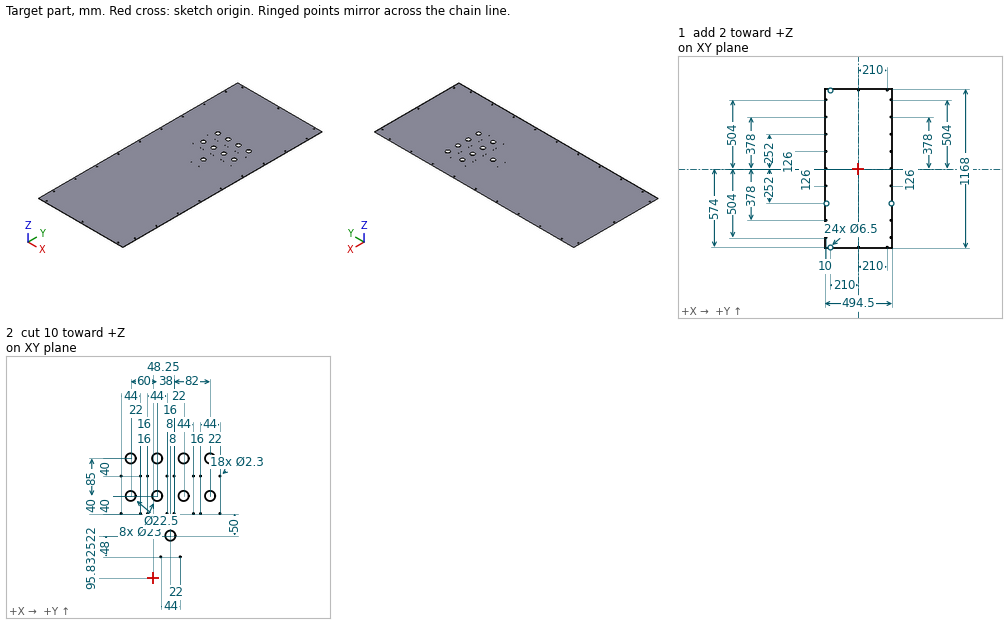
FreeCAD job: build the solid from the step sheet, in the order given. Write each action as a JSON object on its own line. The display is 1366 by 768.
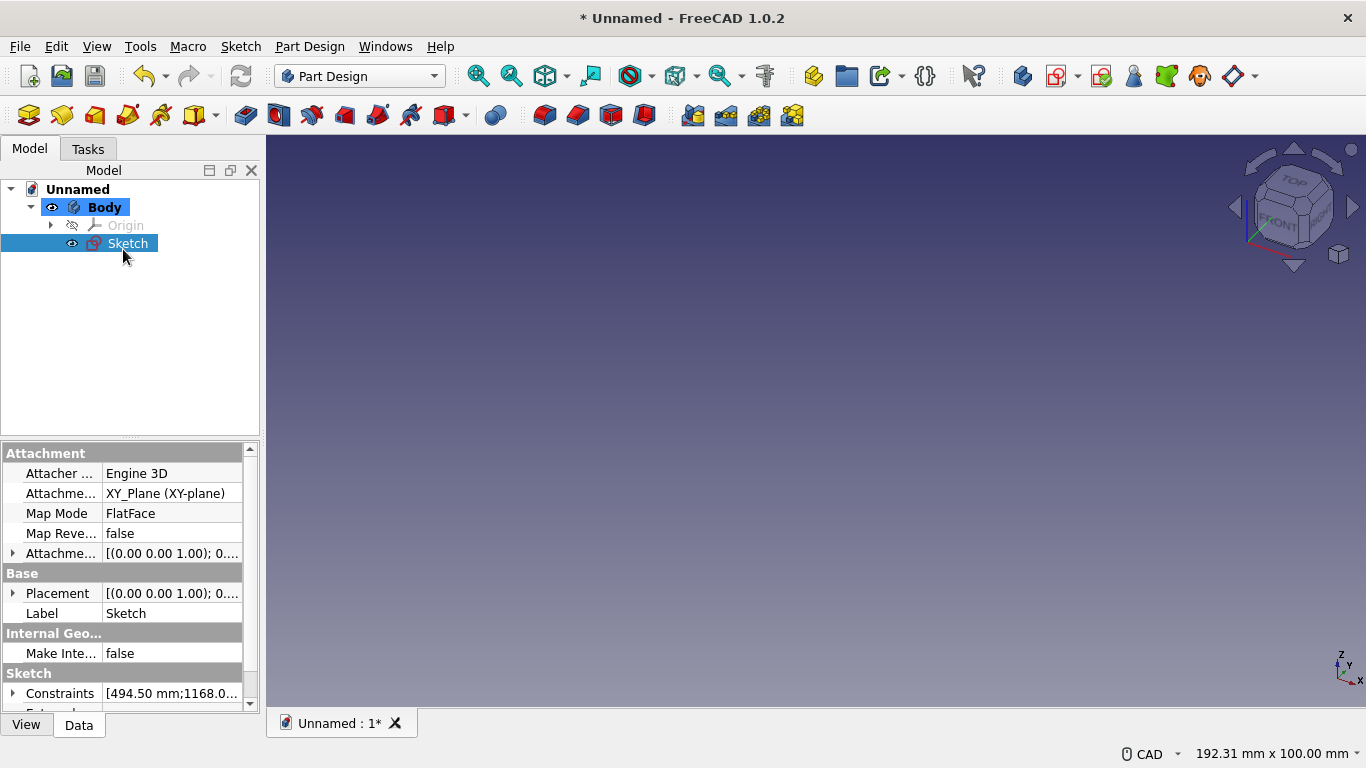
{"action": "left_click", "coordinate": [29, 116]}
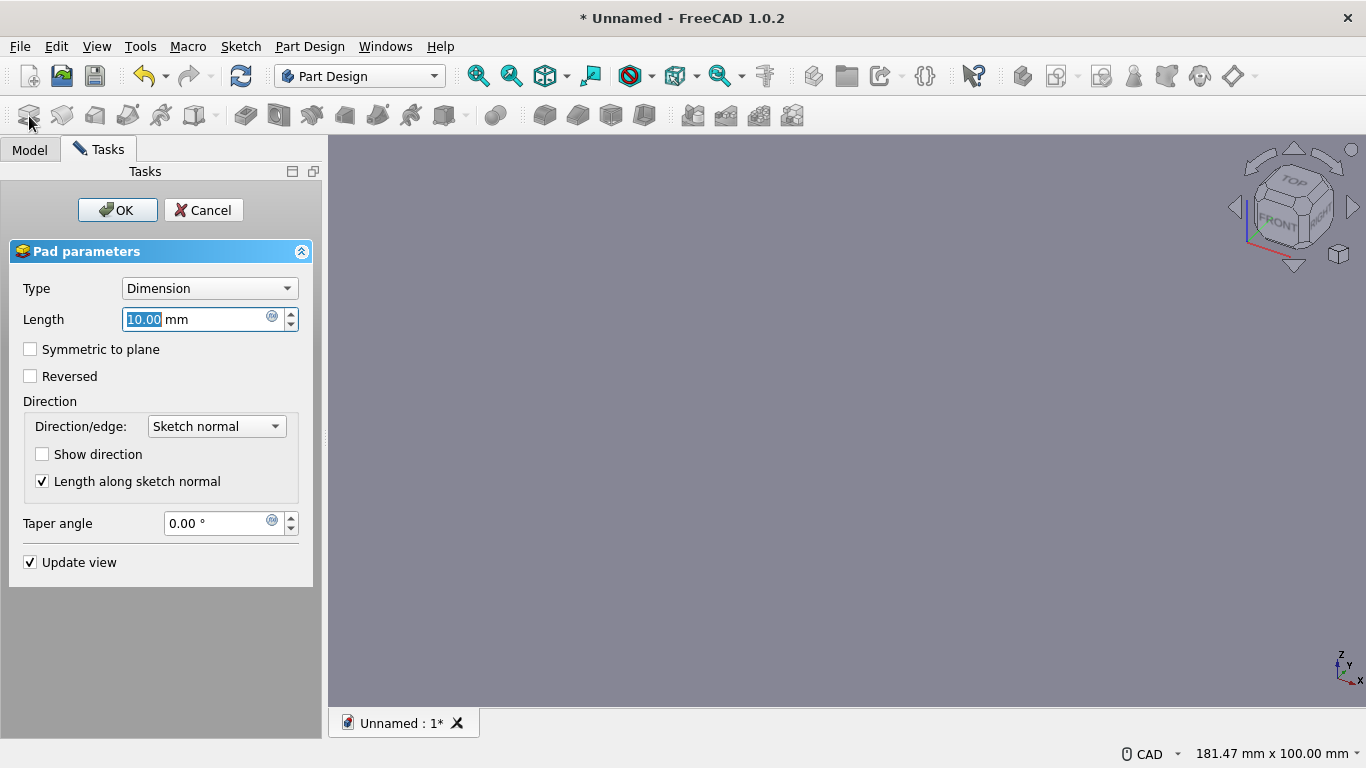
{"action": "type", "text": "2"}
{"action": "key", "text": "Tab"}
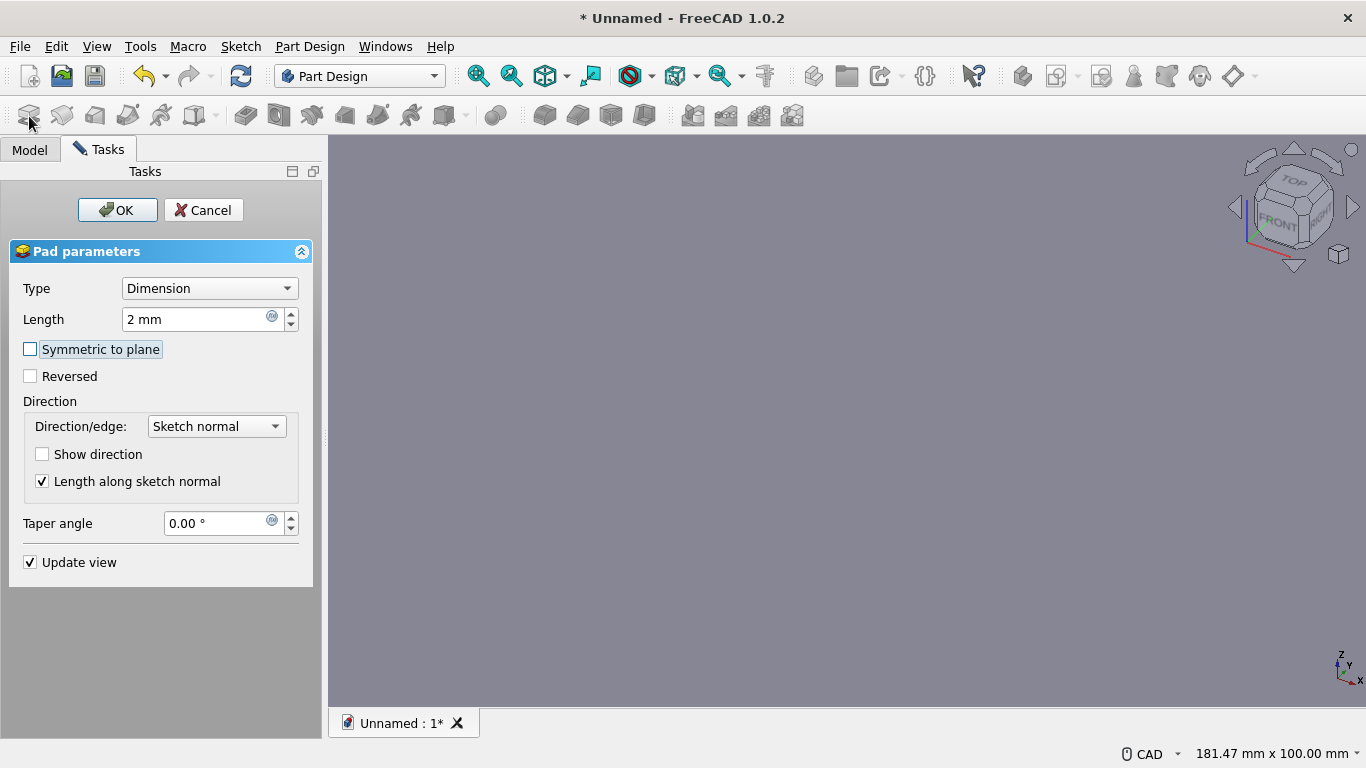
{"action": "left_click", "coordinate": [118, 210]}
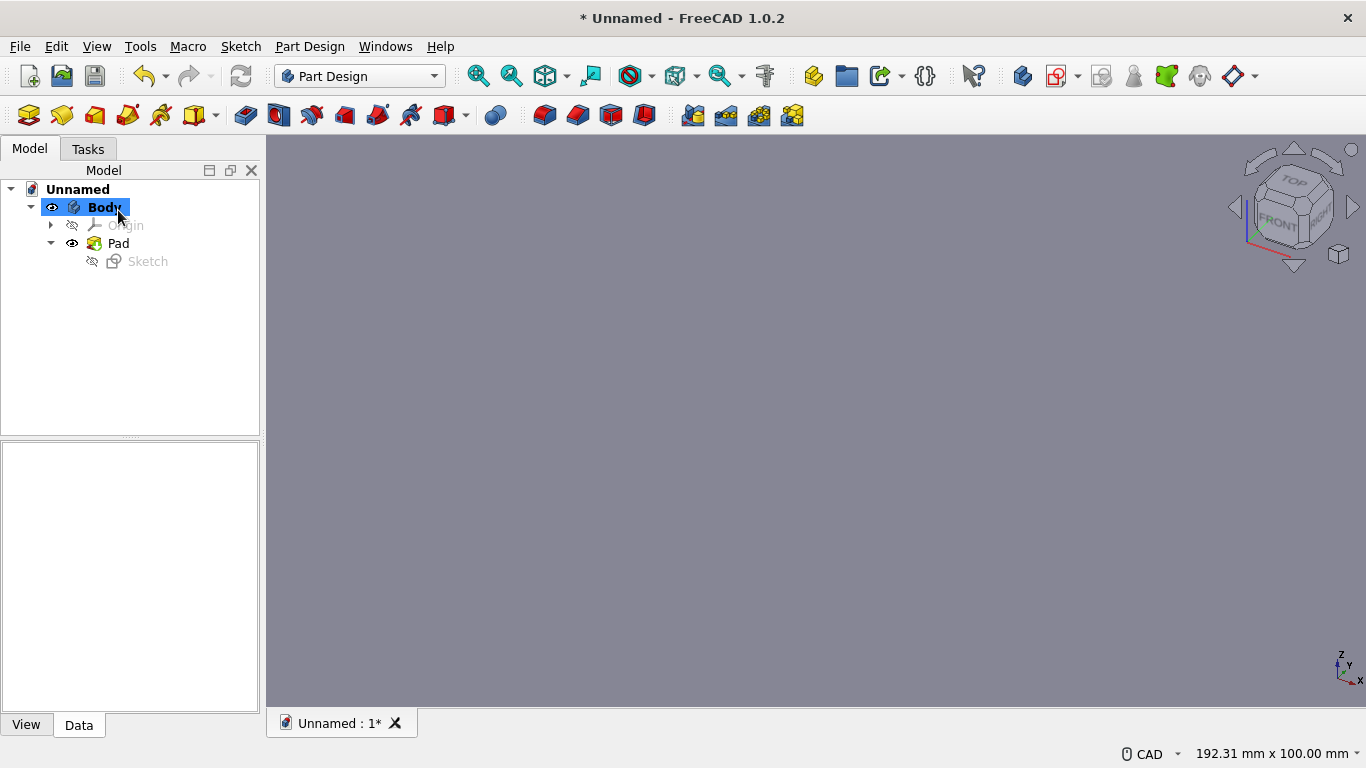
{"action": "left_click", "coordinate": [479, 76]}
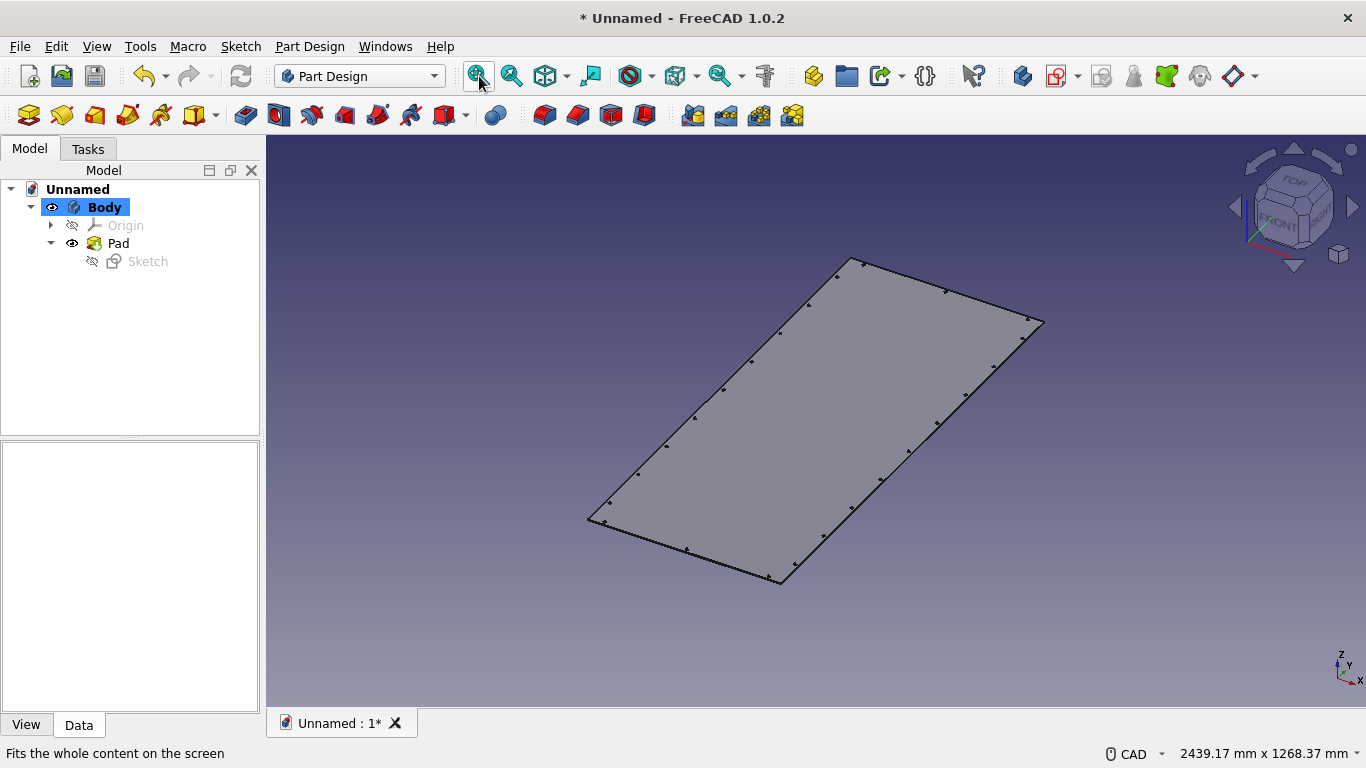
{"action": "left_click", "coordinate": [1056, 76]}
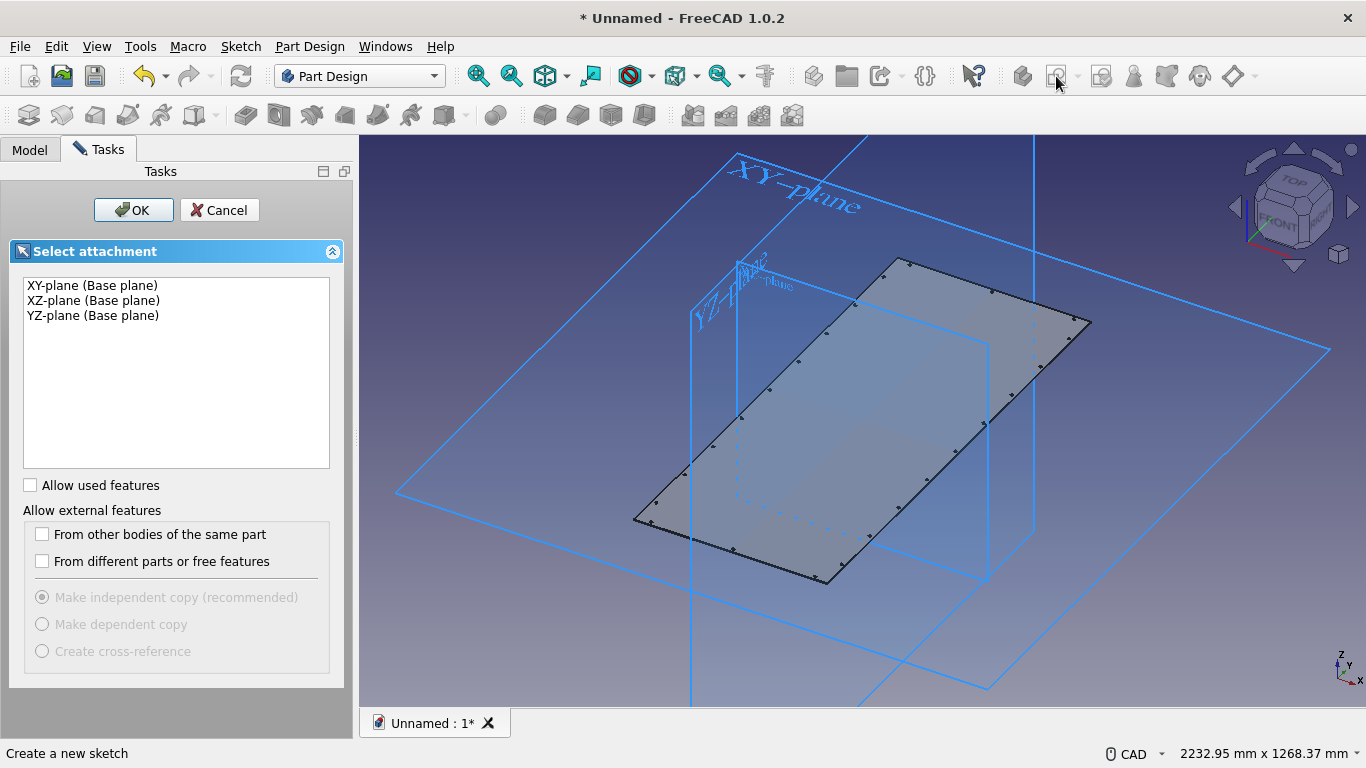
{"action": "left_click", "coordinate": [84, 286]}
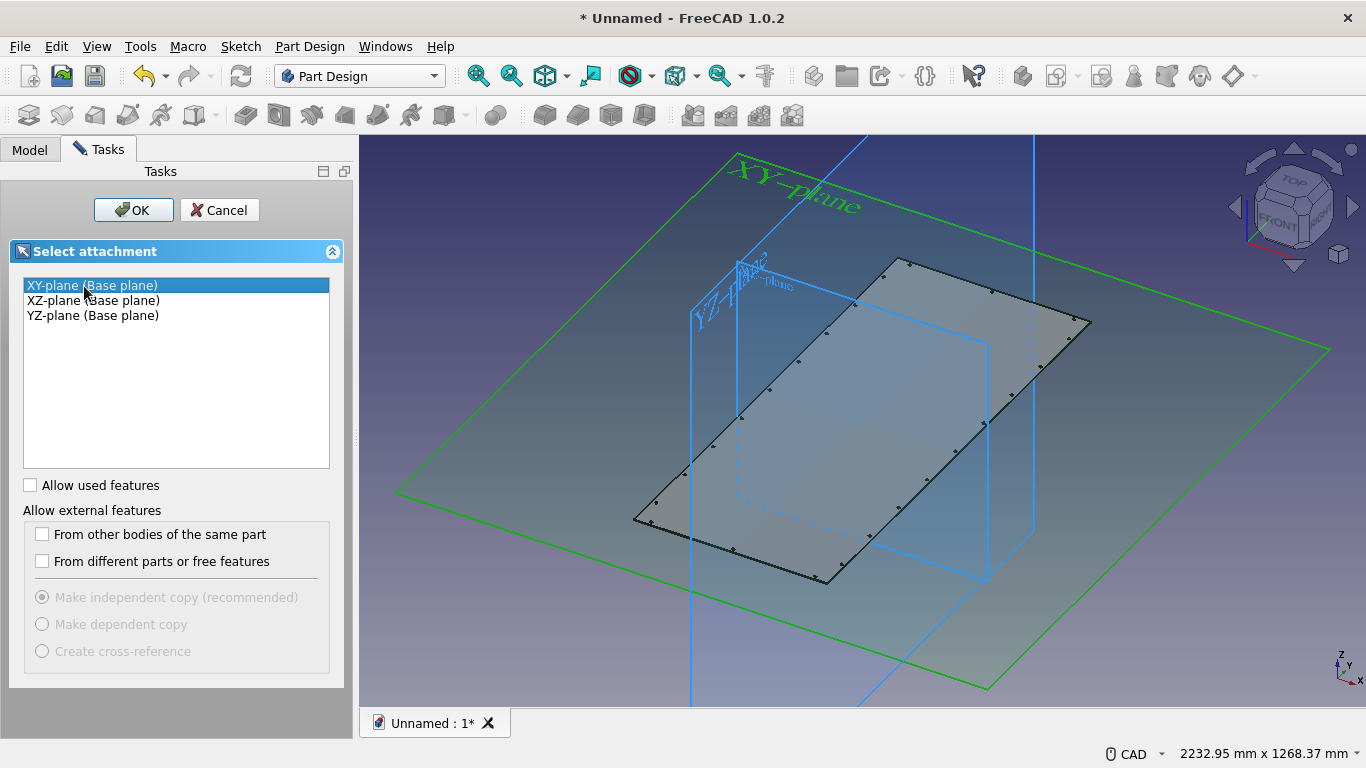
{"action": "left_click", "coordinate": [134, 210]}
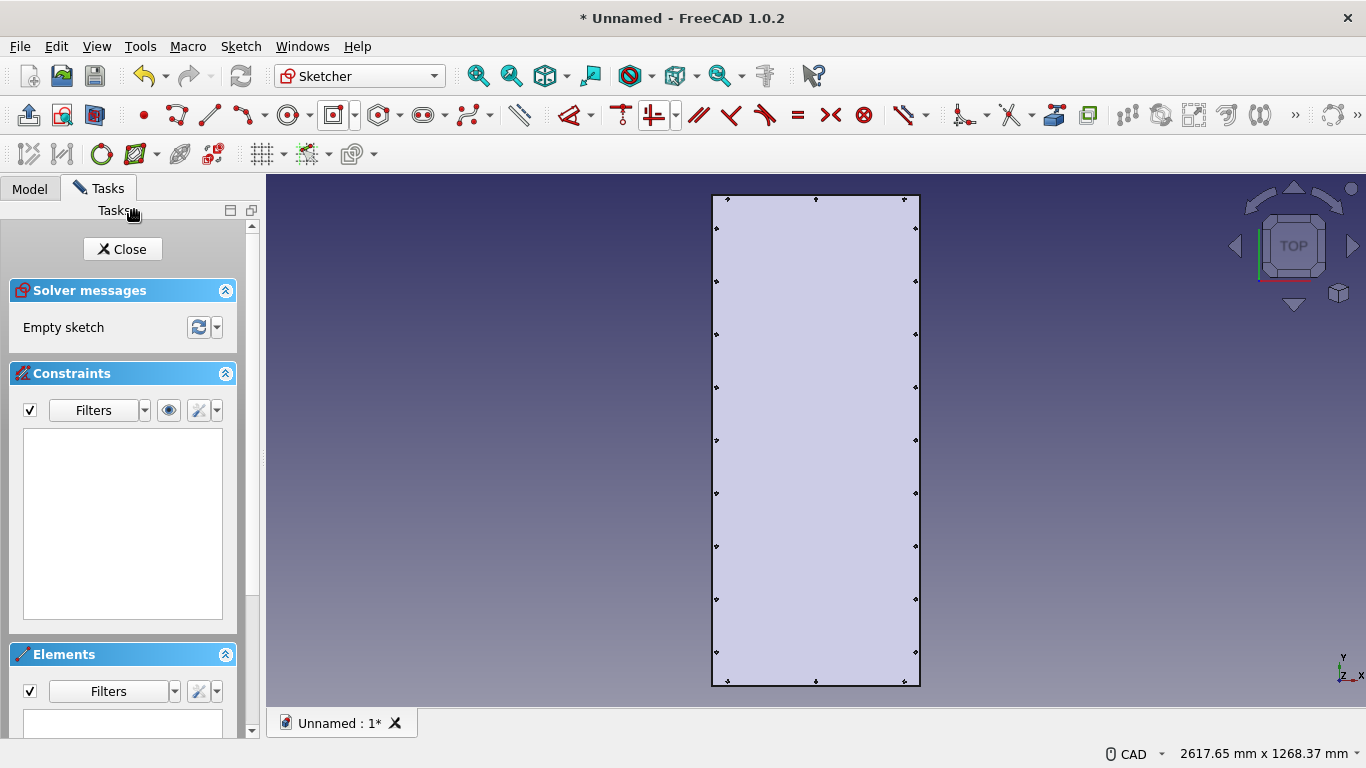
{"action": "left_click", "coordinate": [95, 116]}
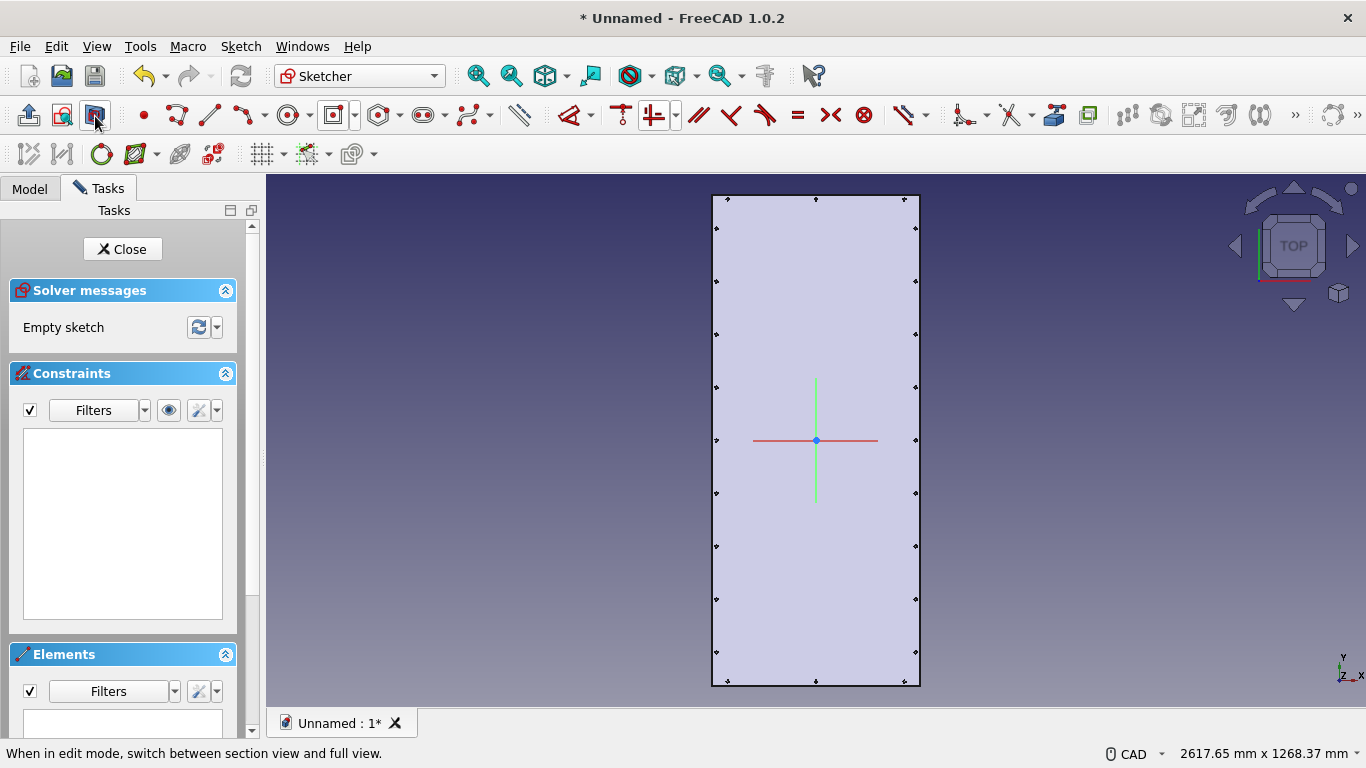
{"action": "scroll", "coordinate": [883, 347], "scroll_direction": "up", "scroll_amount": 5}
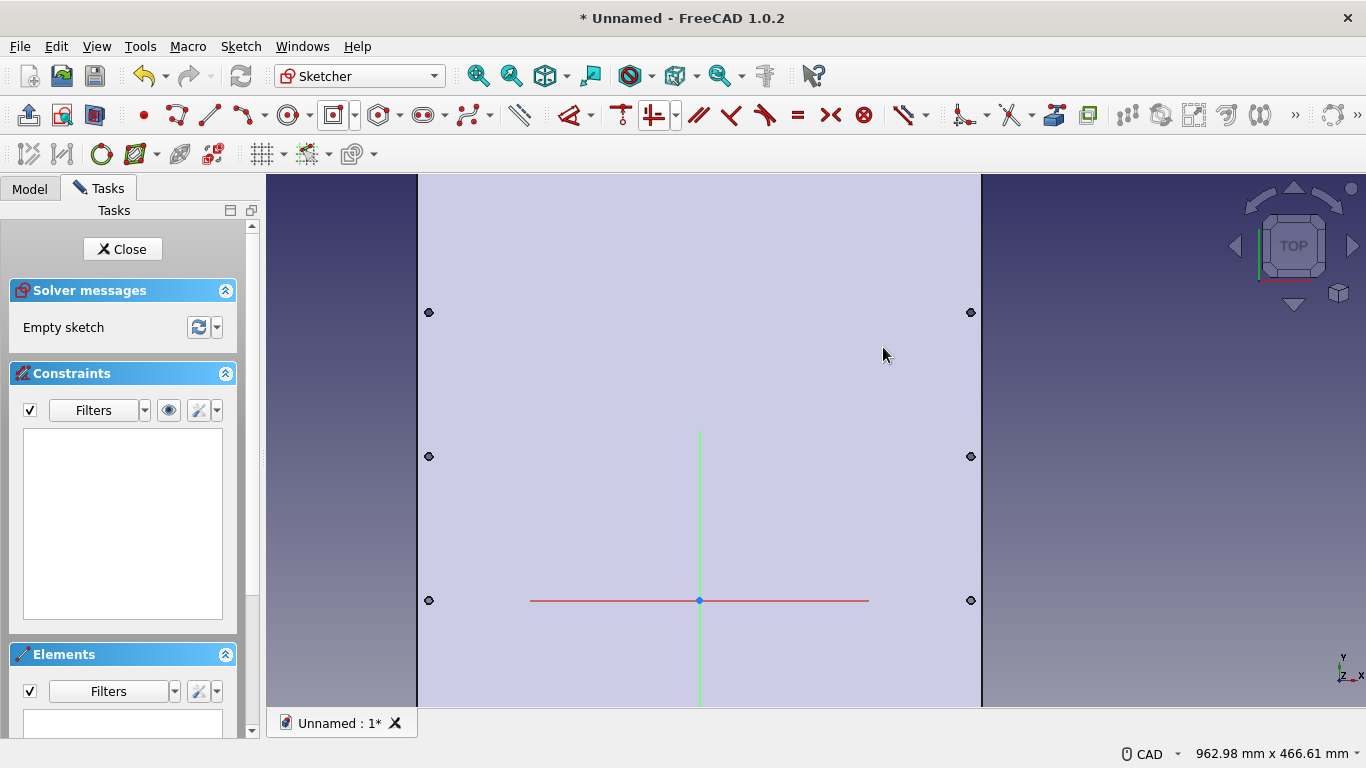
{"action": "left_click", "coordinate": [288, 116]}